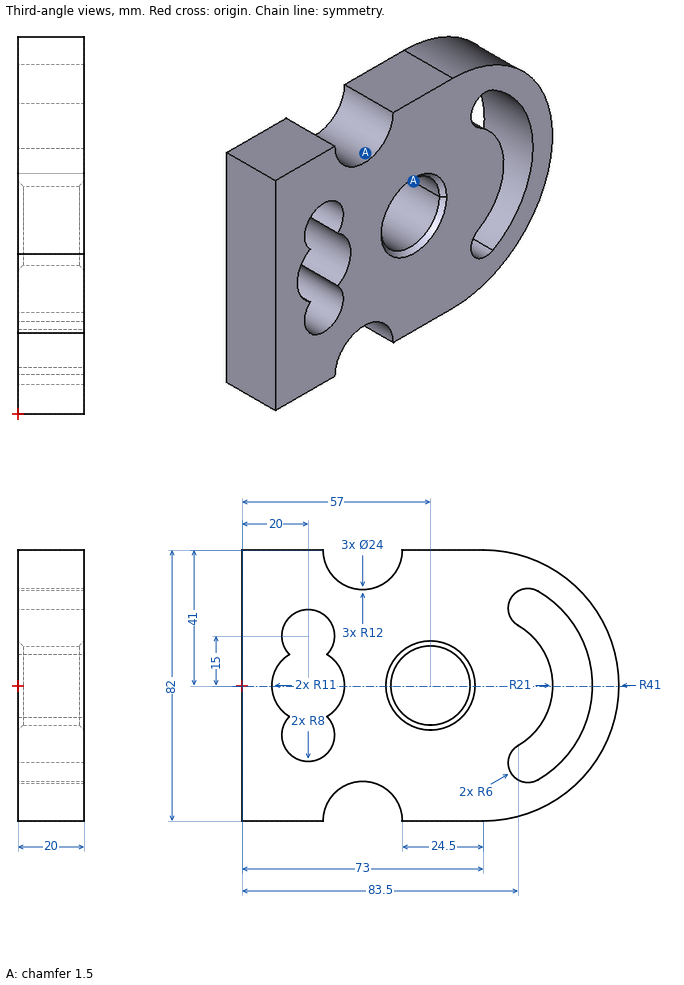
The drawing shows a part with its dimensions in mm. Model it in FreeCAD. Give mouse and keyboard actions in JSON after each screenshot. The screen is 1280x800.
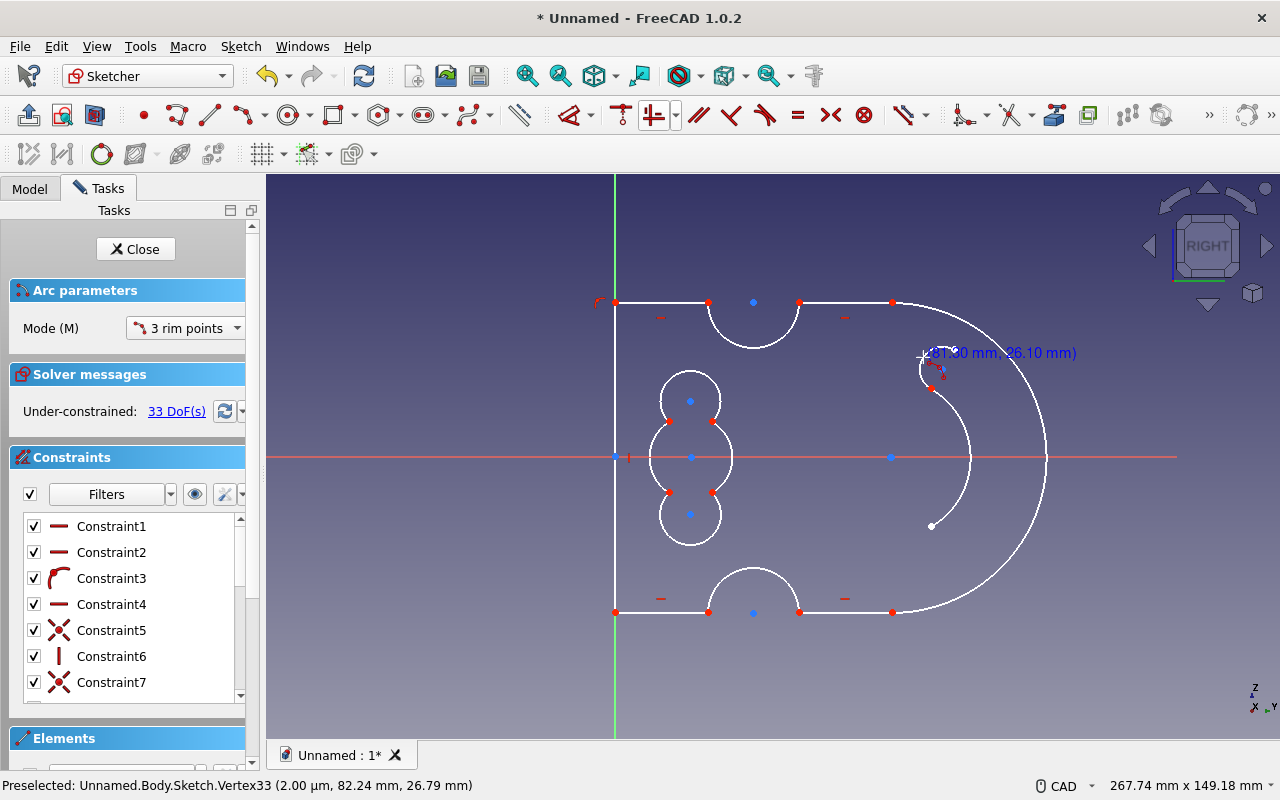
{"action": "left_click", "coordinate": [954, 350]}
{"action": "left_click", "coordinate": [954, 565]}
{"action": "left_click", "coordinate": [1014, 483]}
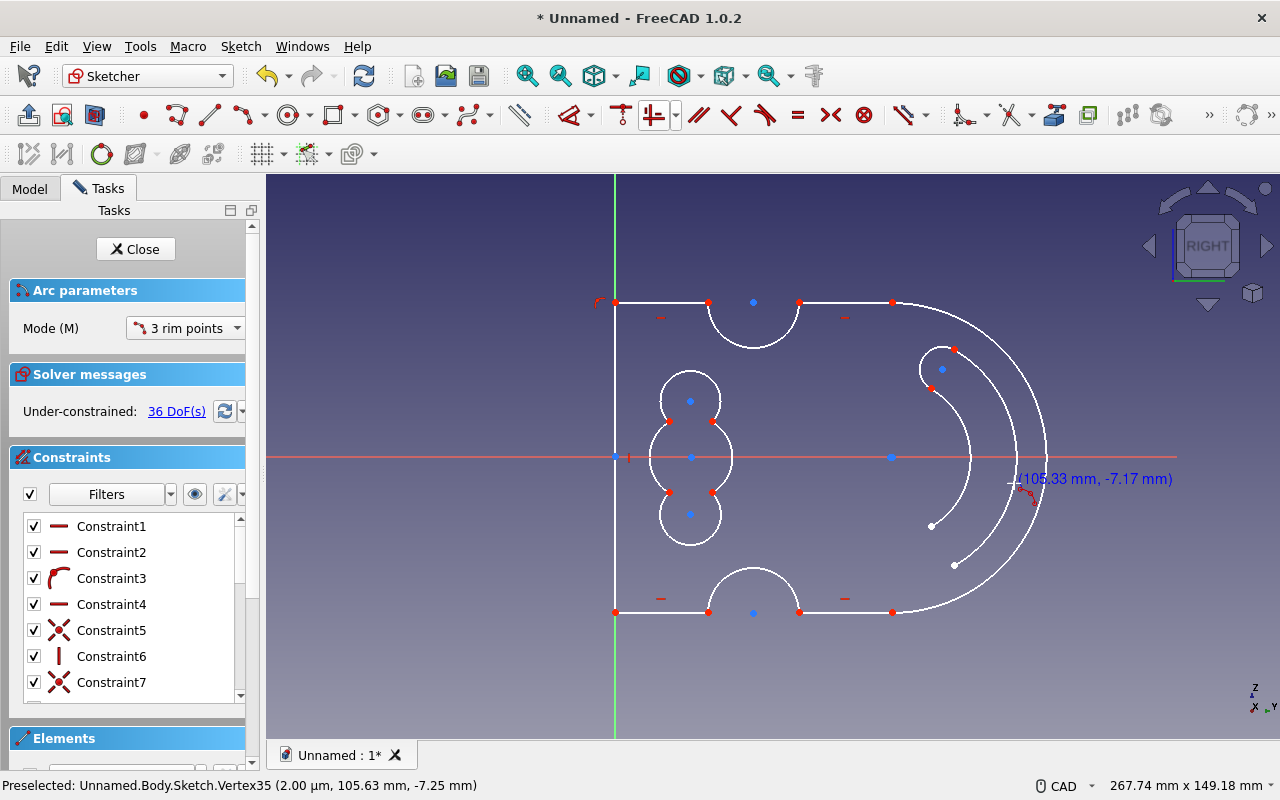
{"action": "left_click", "coordinate": [954, 566]}
{"action": "left_click", "coordinate": [931, 527]}
{"action": "left_click", "coordinate": [923, 557]}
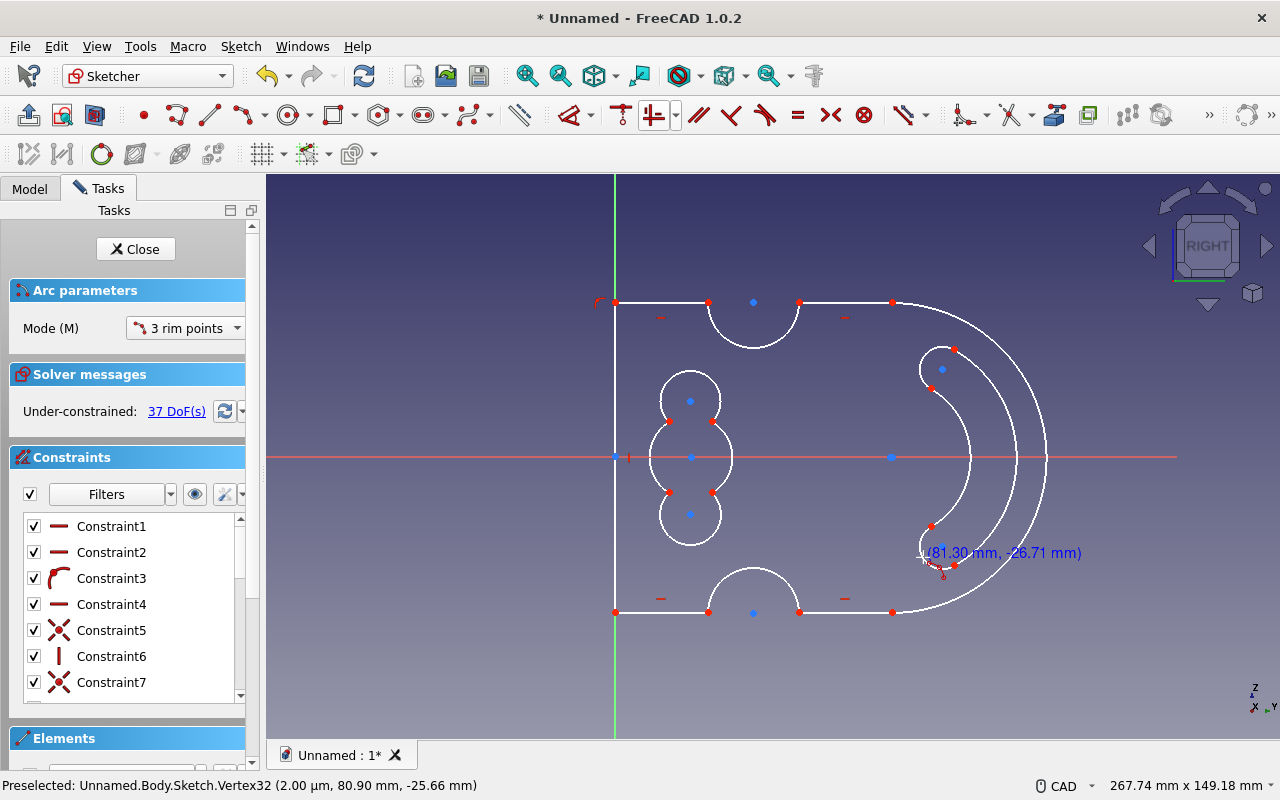
{"action": "key", "text": "g c"}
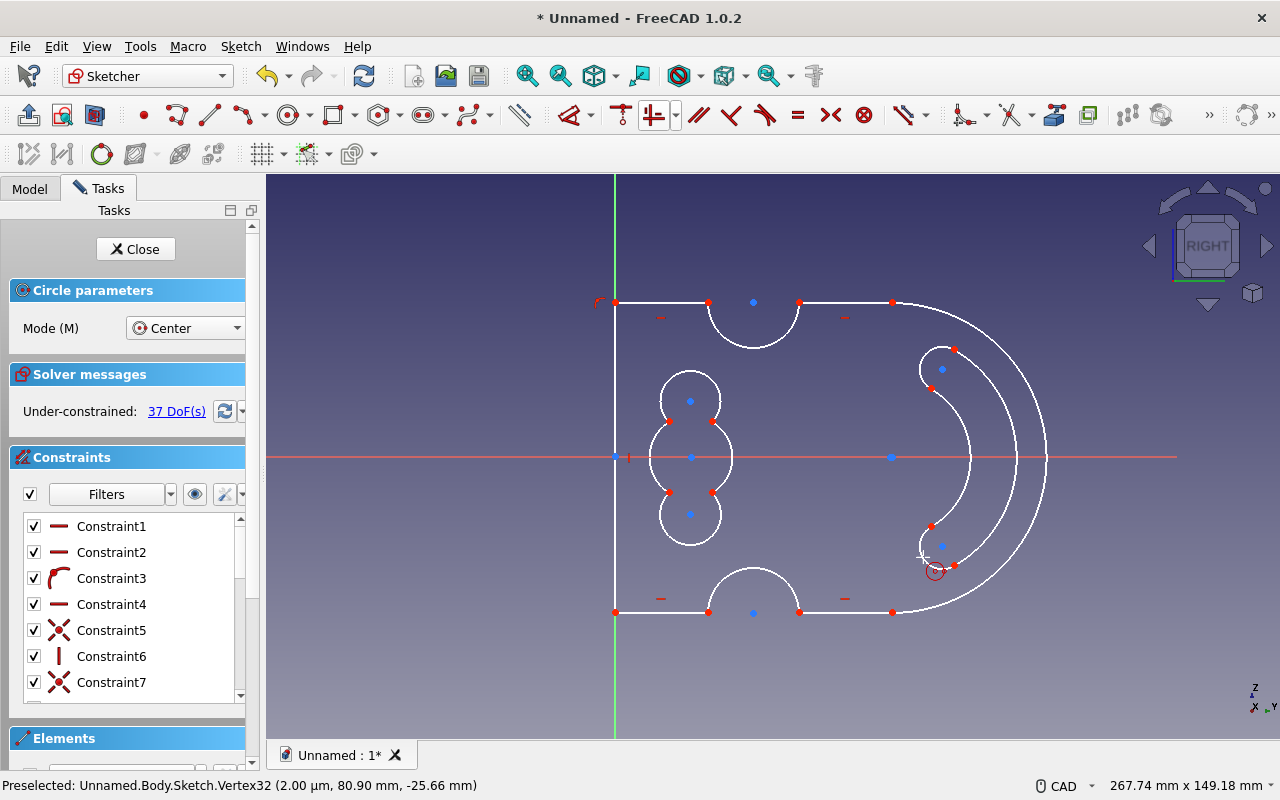
{"action": "left_click", "coordinate": [831, 457]}
{"action": "left_click", "coordinate": [863, 425]}
{"action": "key", "text": "Escape"}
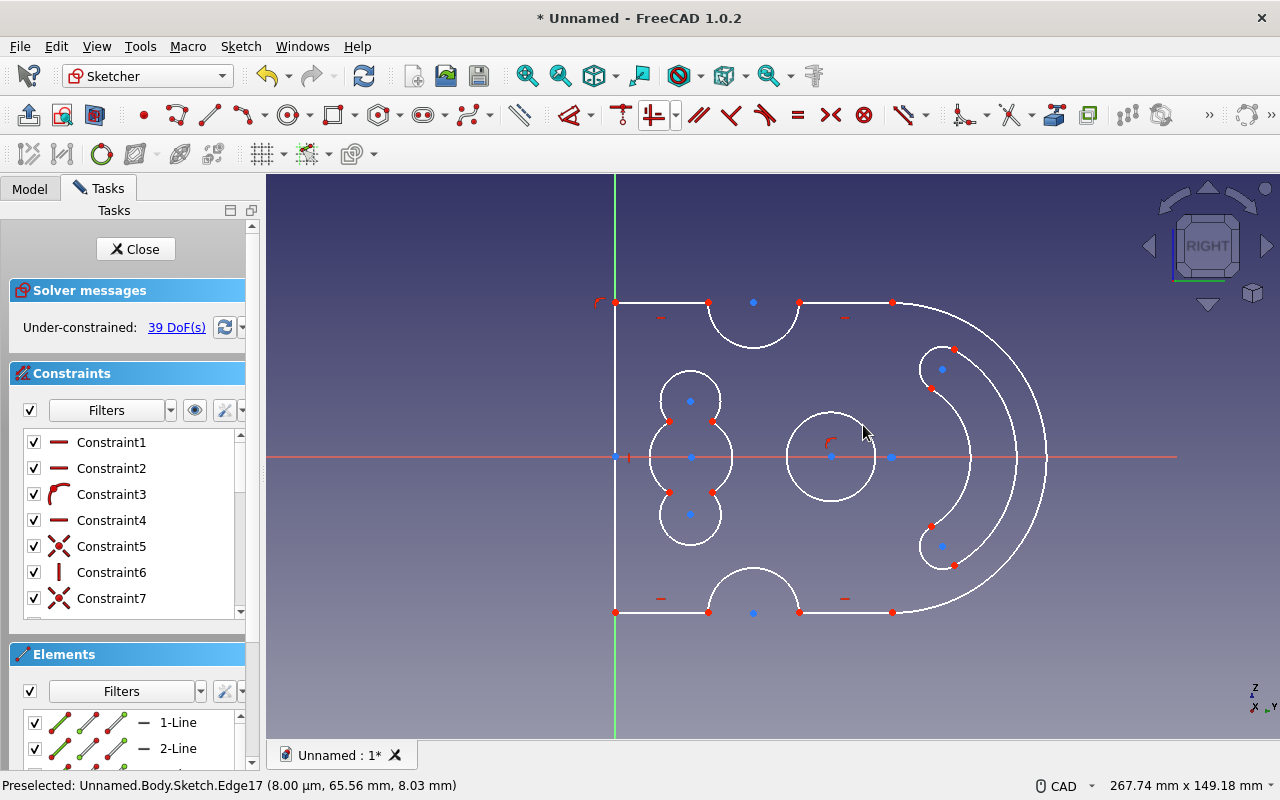
{"action": "left_click", "coordinate": [964, 490]}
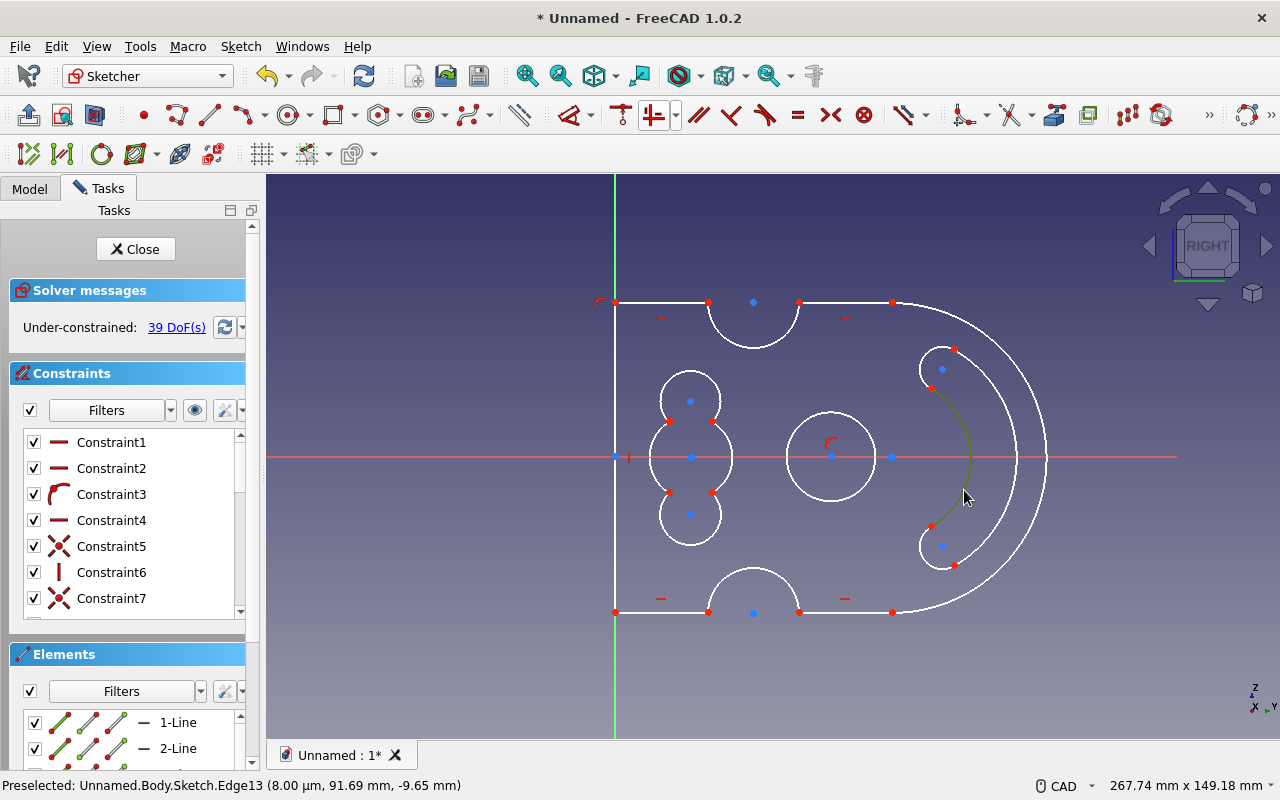
{"action": "left_click", "coordinate": [933, 349]}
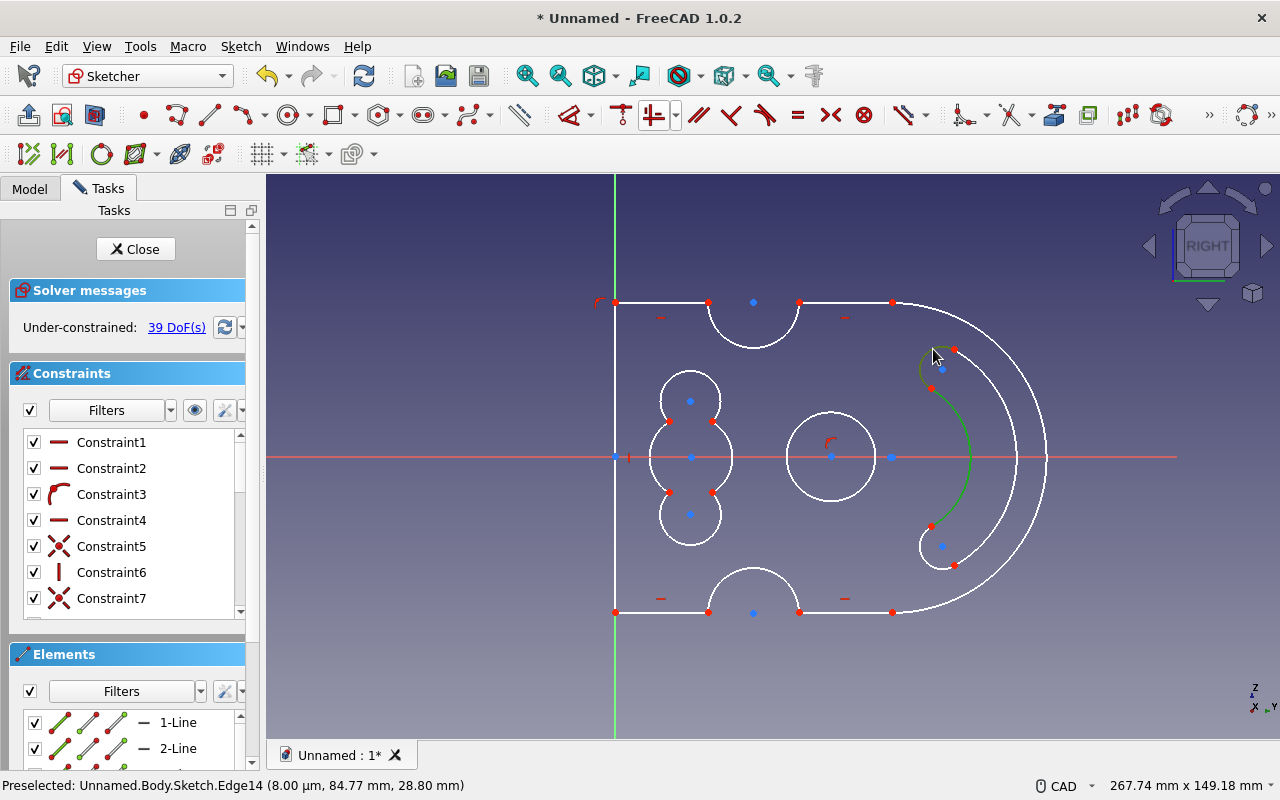
{"action": "key", "text": "t"}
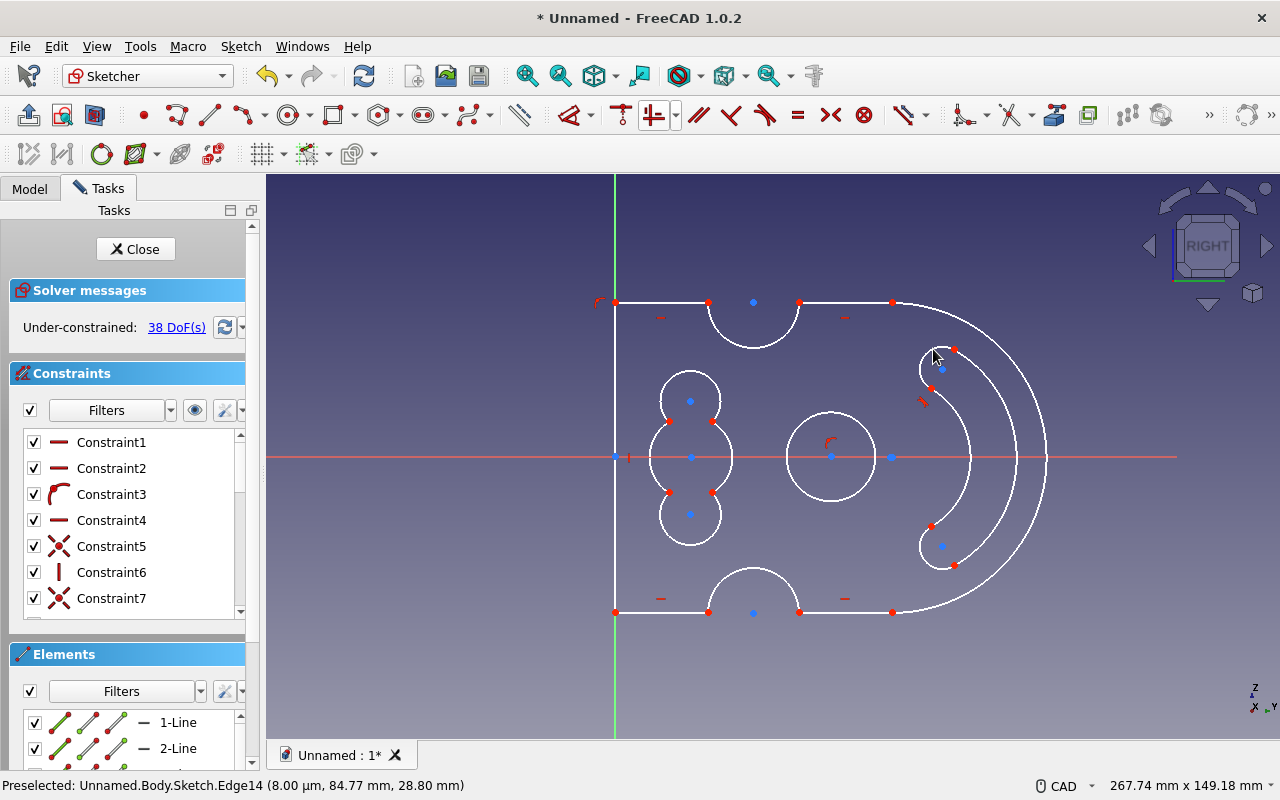
{"action": "left_click", "coordinate": [964, 490]}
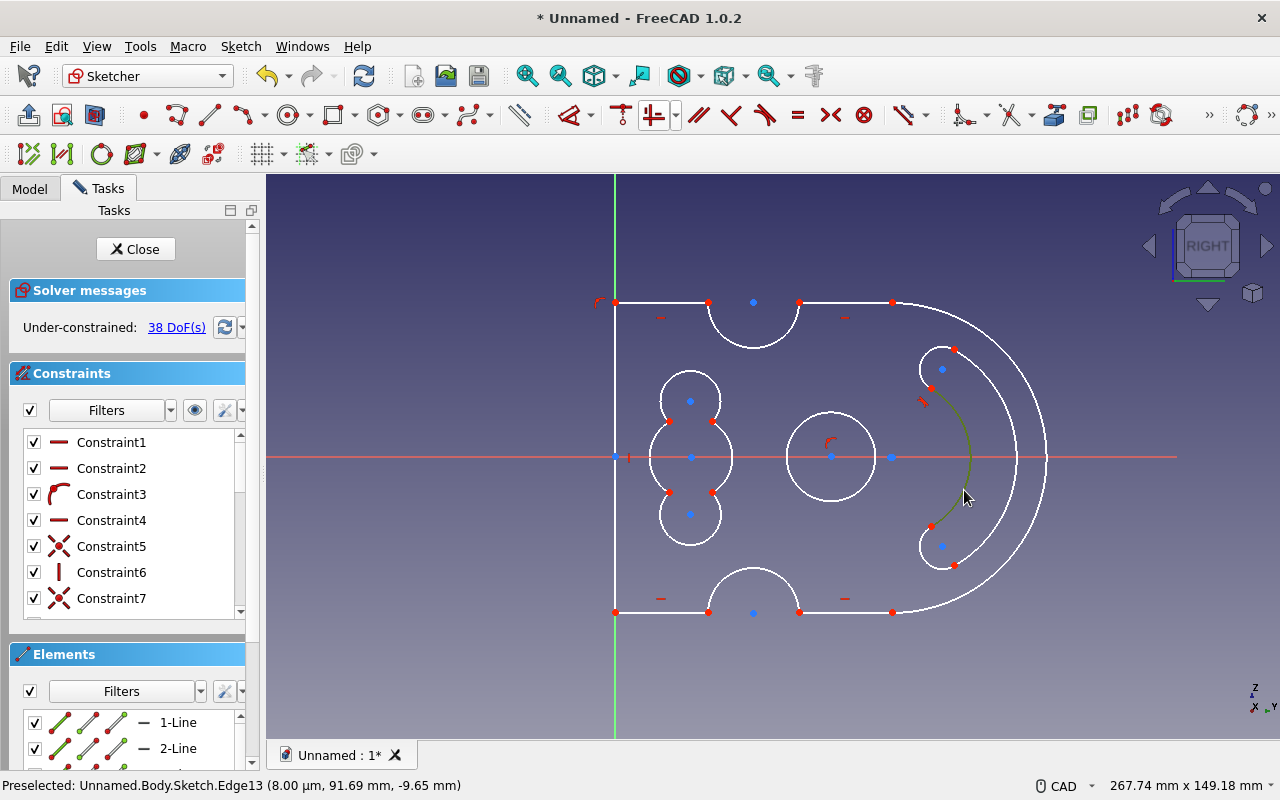
{"action": "left_click", "coordinate": [920, 544]}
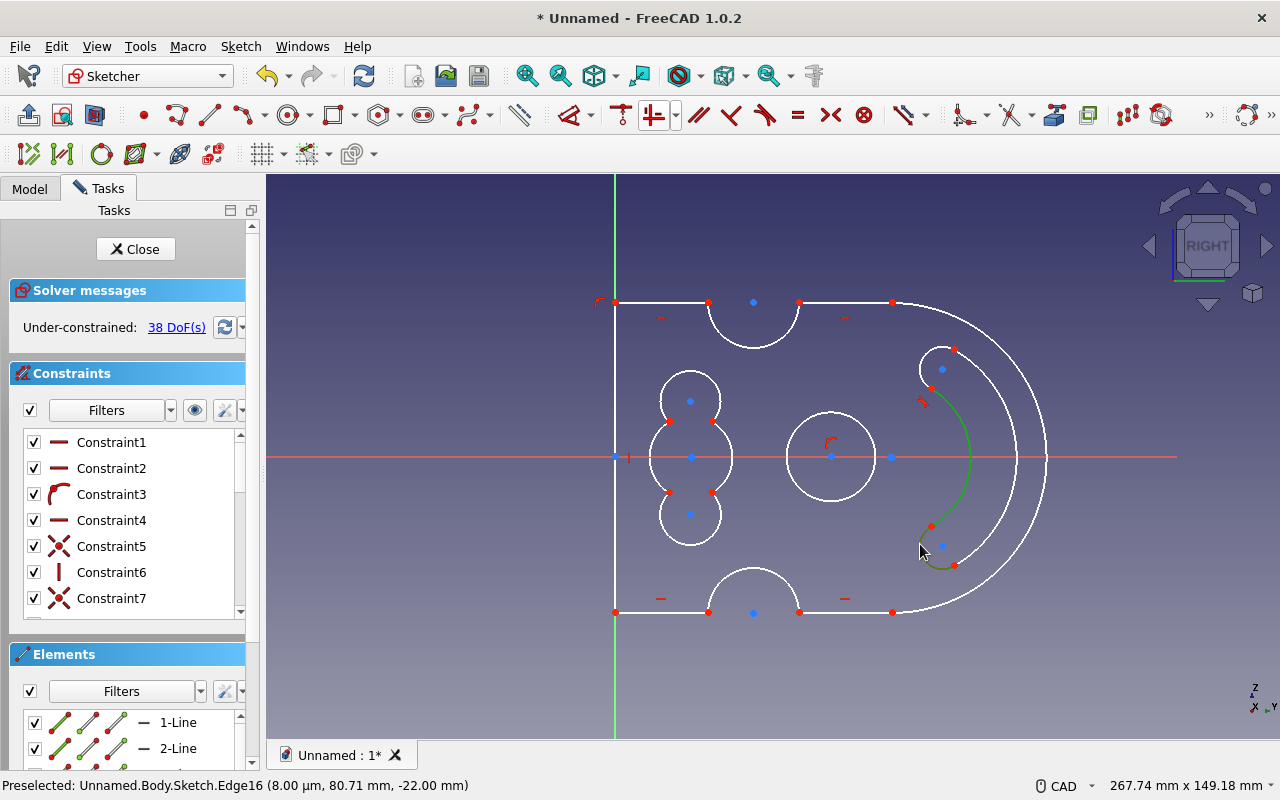
{"action": "left_click", "coordinate": [765, 116]}